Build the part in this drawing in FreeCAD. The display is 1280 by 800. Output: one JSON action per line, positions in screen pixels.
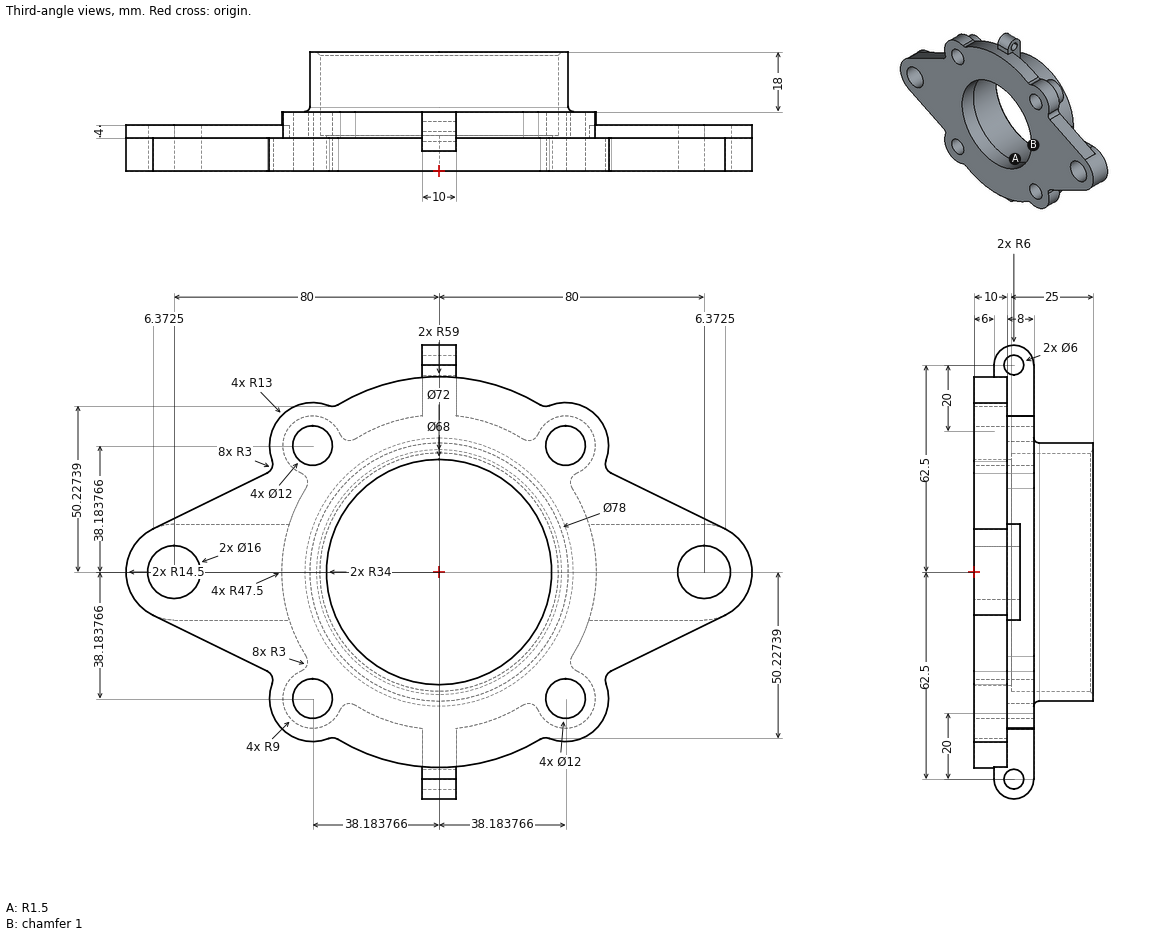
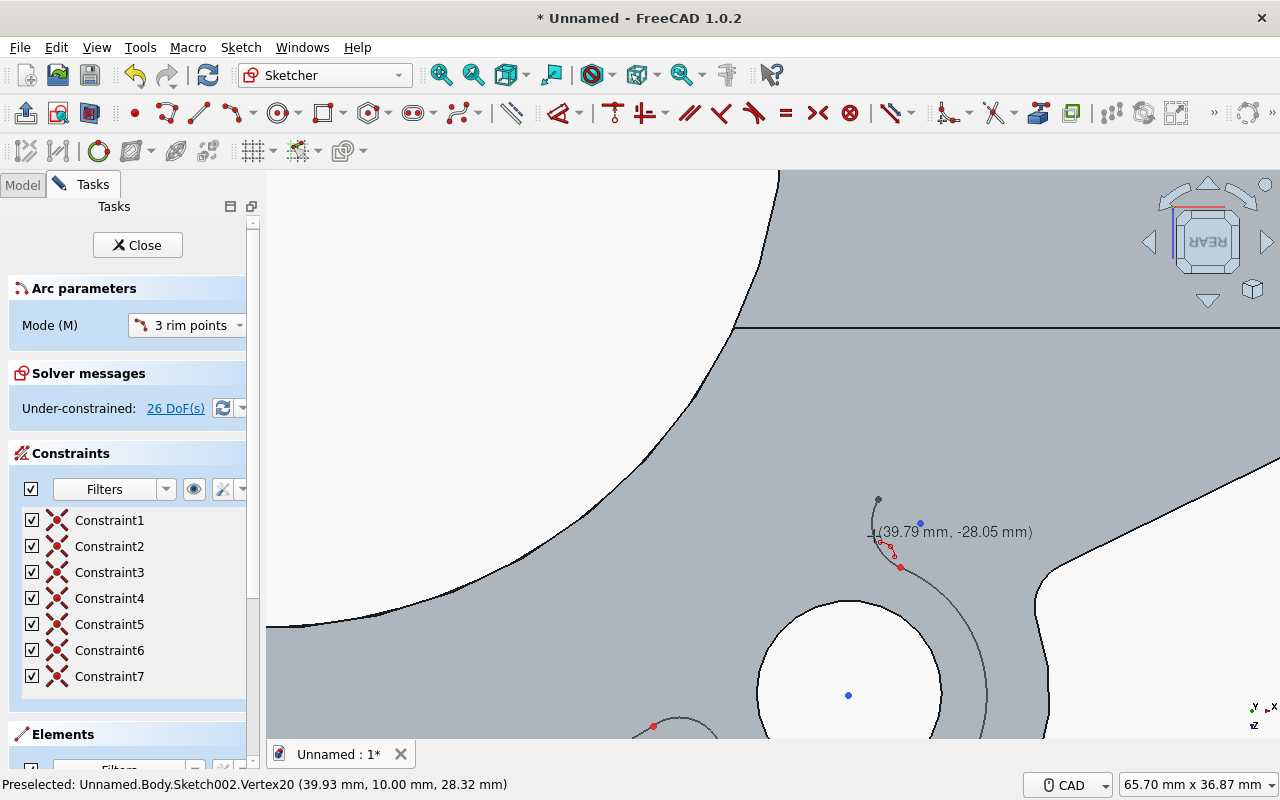
{"action": "scroll", "coordinate": [850, 569], "scroll_direction": "down", "scroll_amount": 7}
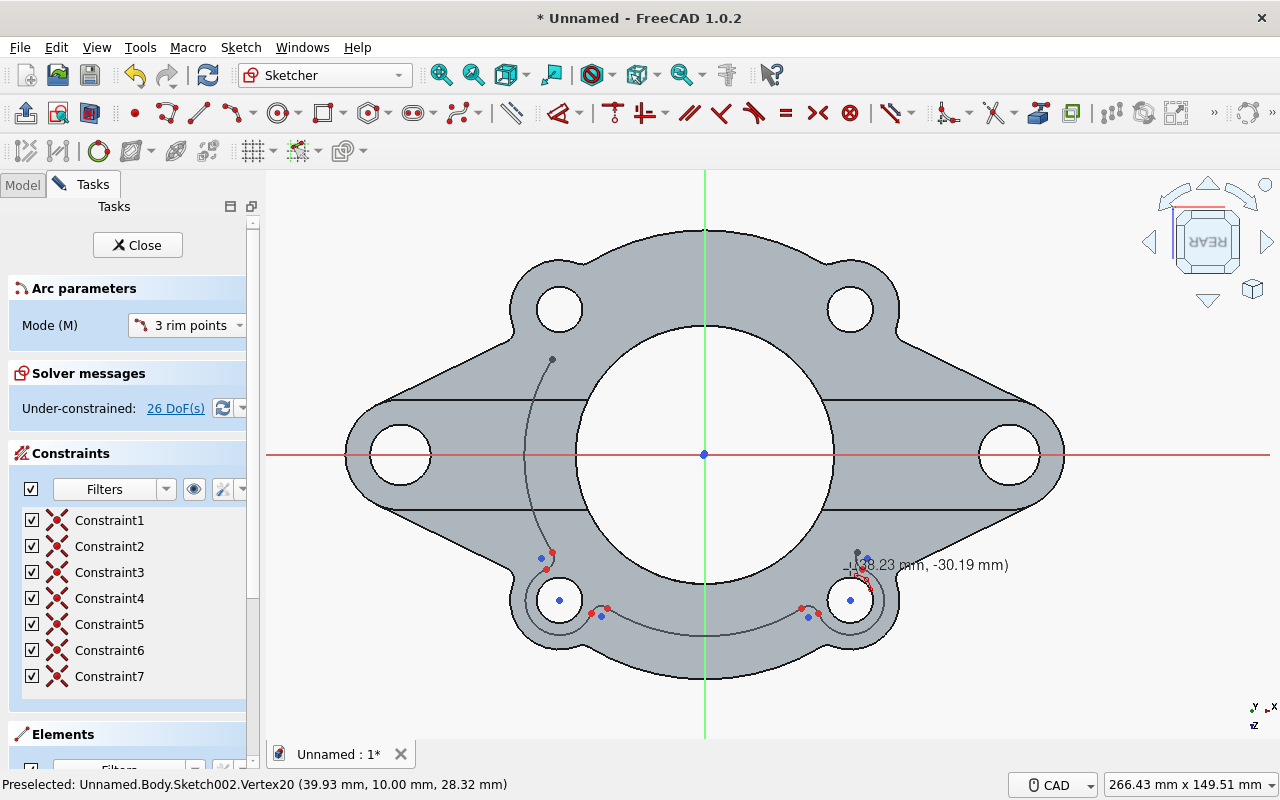
{"action": "scroll", "coordinate": [858, 552], "scroll_direction": "up", "scroll_amount": 2}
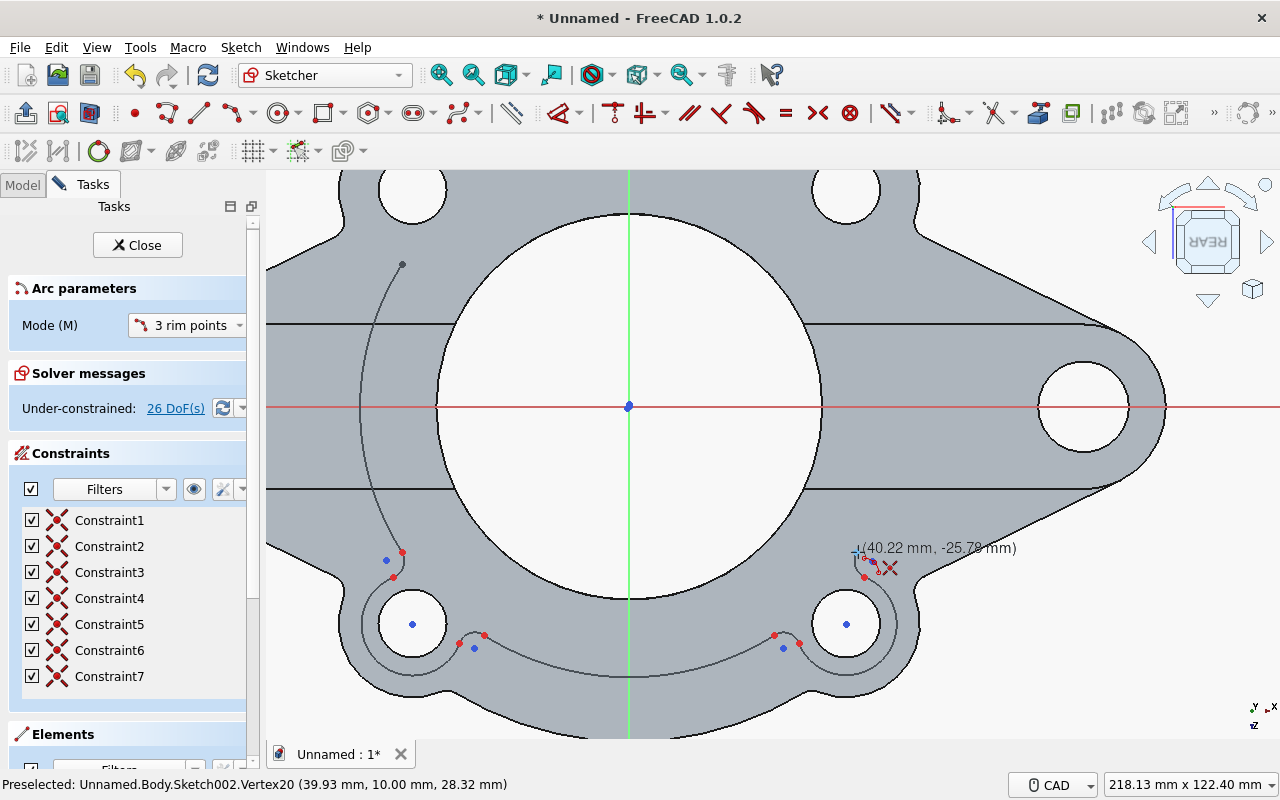
{"action": "left_click", "coordinate": [857, 552]}
{"action": "left_click", "coordinate": [857, 262]}
{"action": "left_click", "coordinate": [897, 437]}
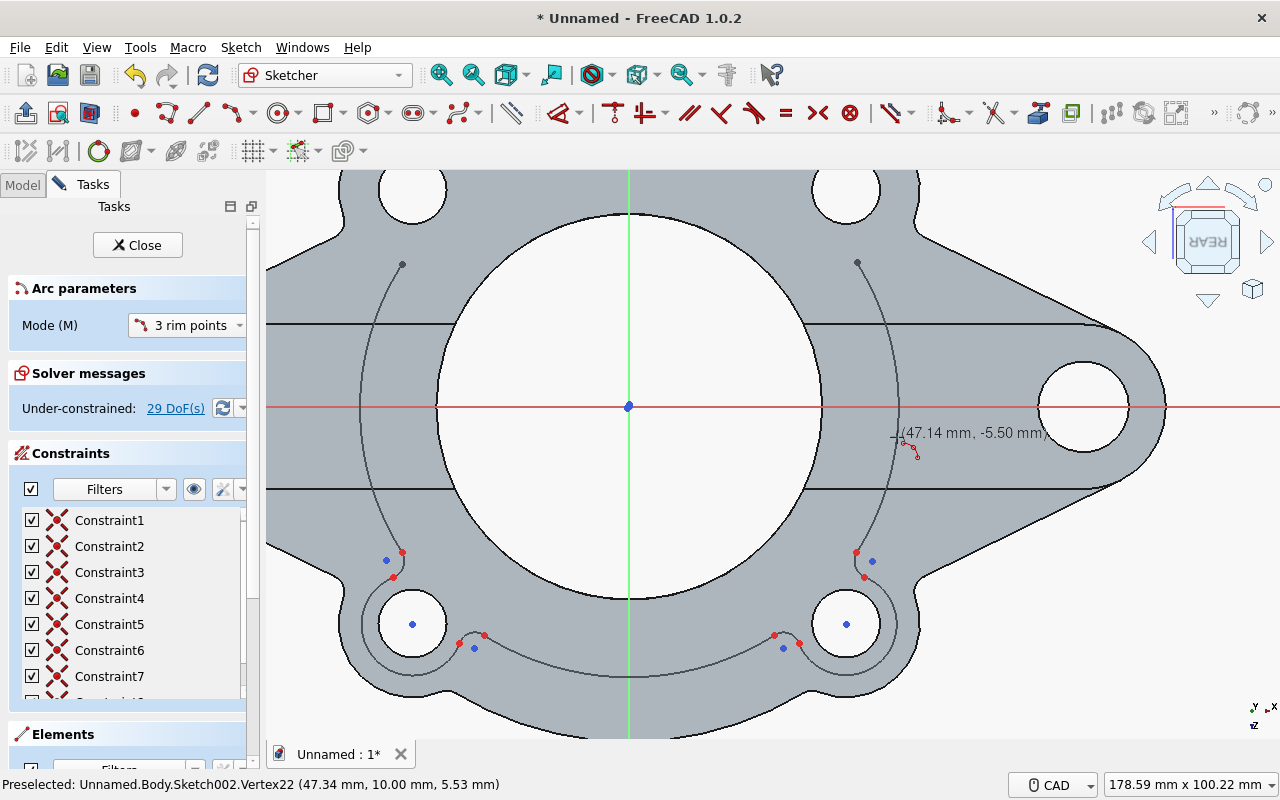
{"action": "left_click", "coordinate": [857, 263]}
{"action": "left_click", "coordinate": [865, 237]}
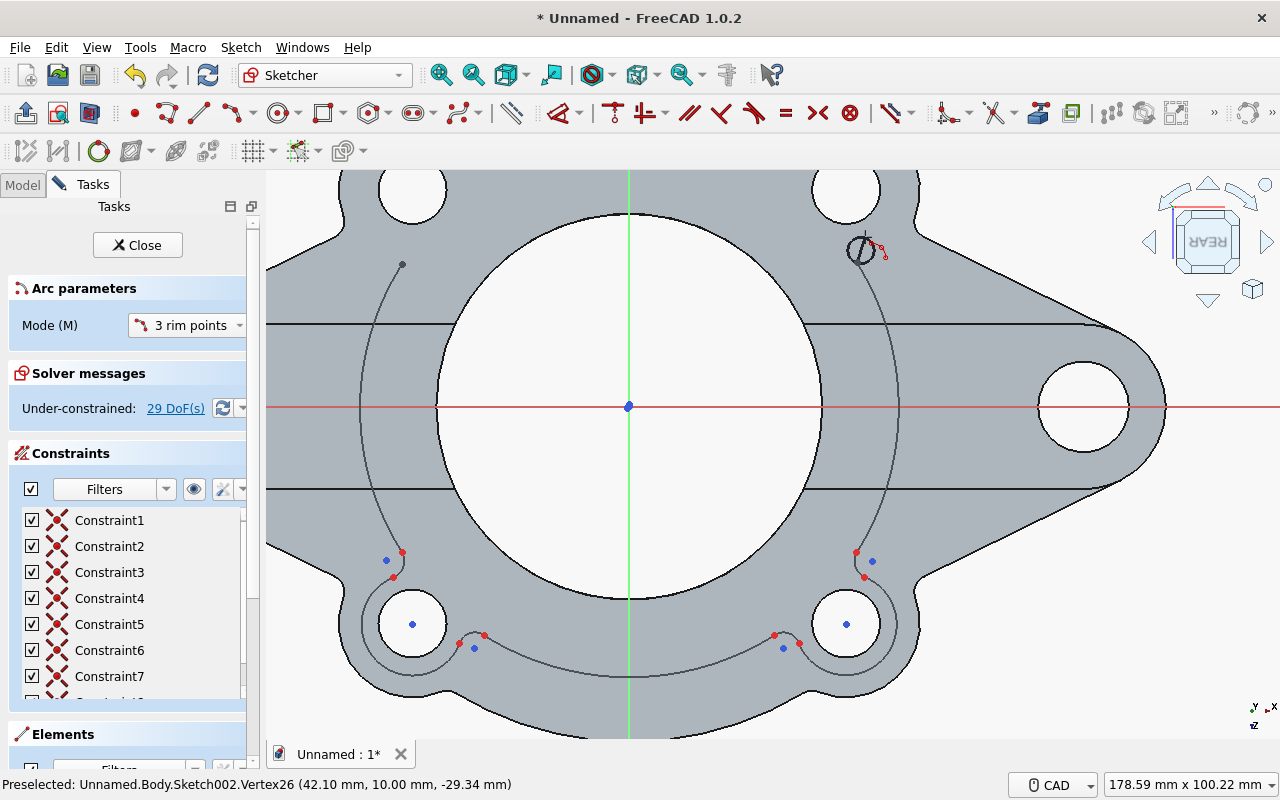
{"action": "scroll", "coordinate": [855, 248], "scroll_direction": "up", "scroll_amount": 5}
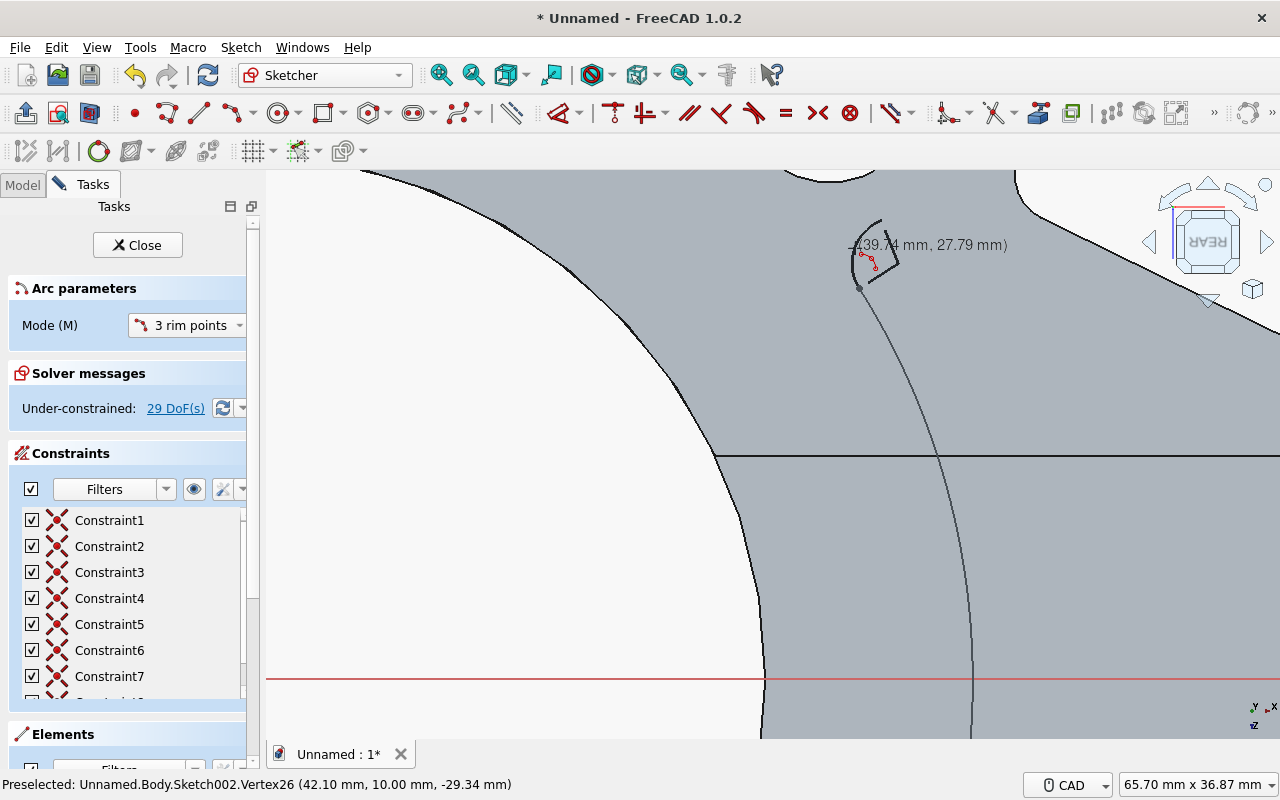
{"action": "left_click", "coordinate": [855, 248]}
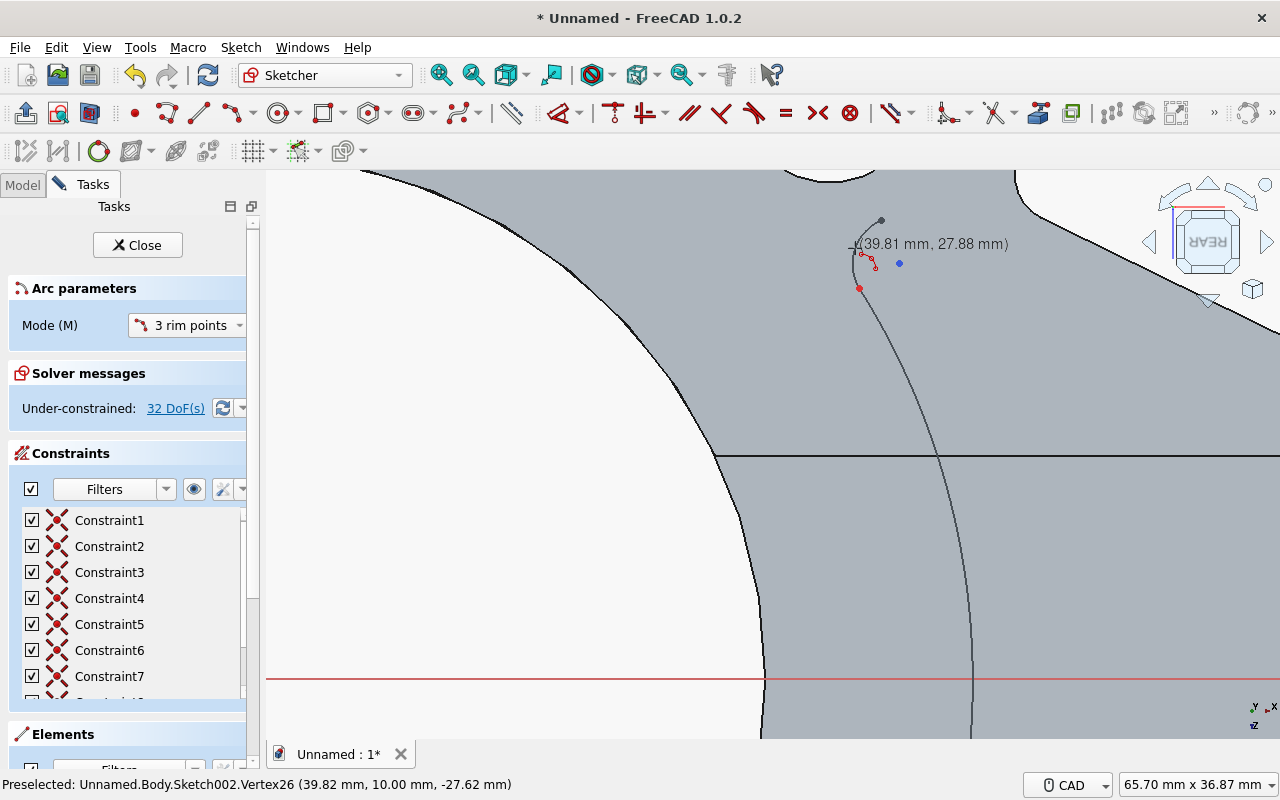
{"action": "scroll", "coordinate": [856, 381], "scroll_direction": "down", "scroll_amount": 7}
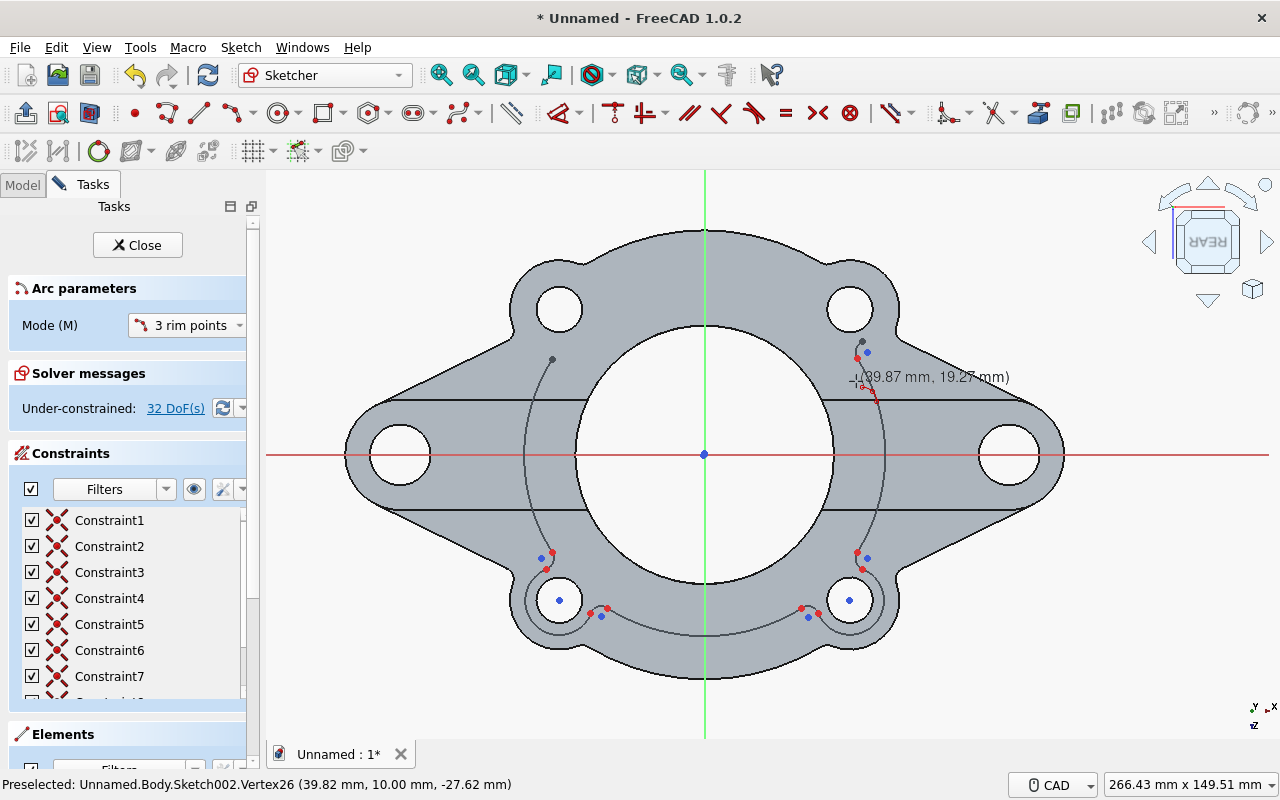
{"action": "scroll", "coordinate": [863, 341], "scroll_direction": "up", "scroll_amount": 2}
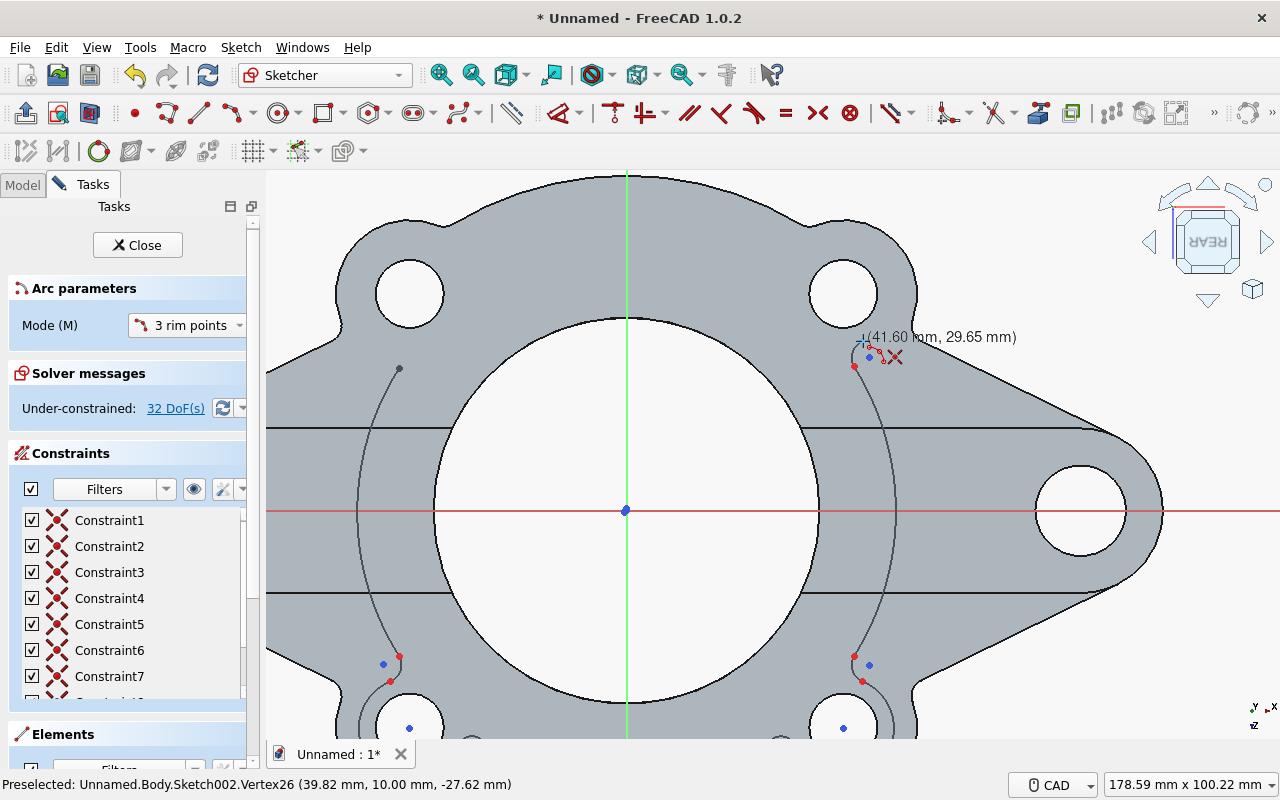
{"action": "left_click", "coordinate": [862, 342]}
{"action": "left_click", "coordinate": [796, 275]}
{"action": "left_click", "coordinate": [879, 258]}